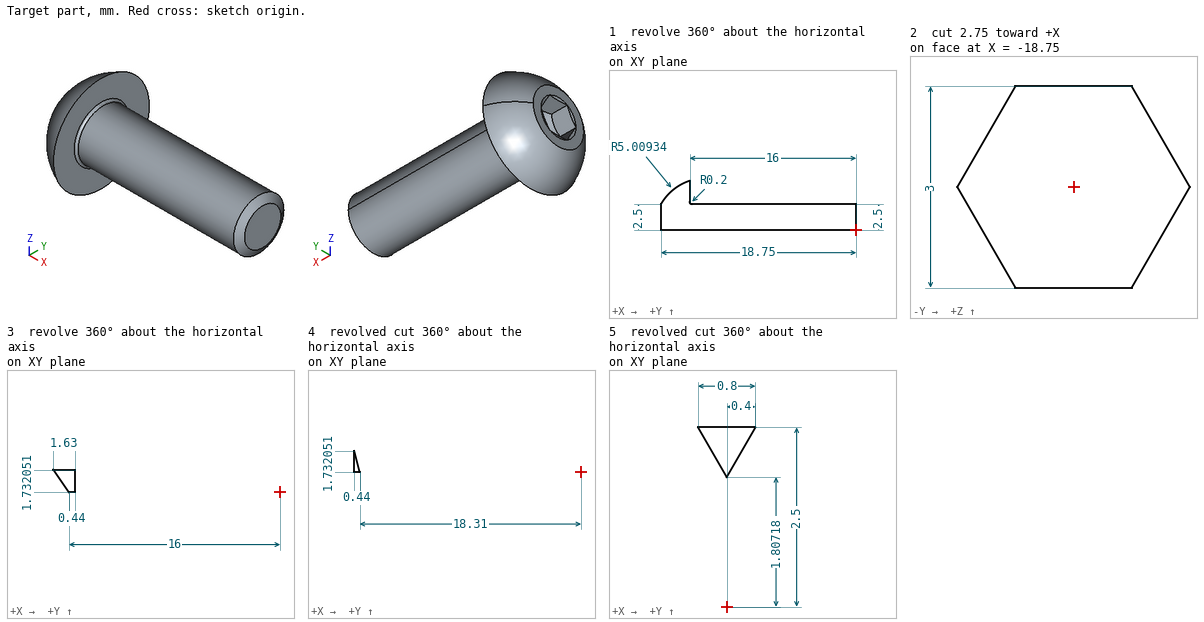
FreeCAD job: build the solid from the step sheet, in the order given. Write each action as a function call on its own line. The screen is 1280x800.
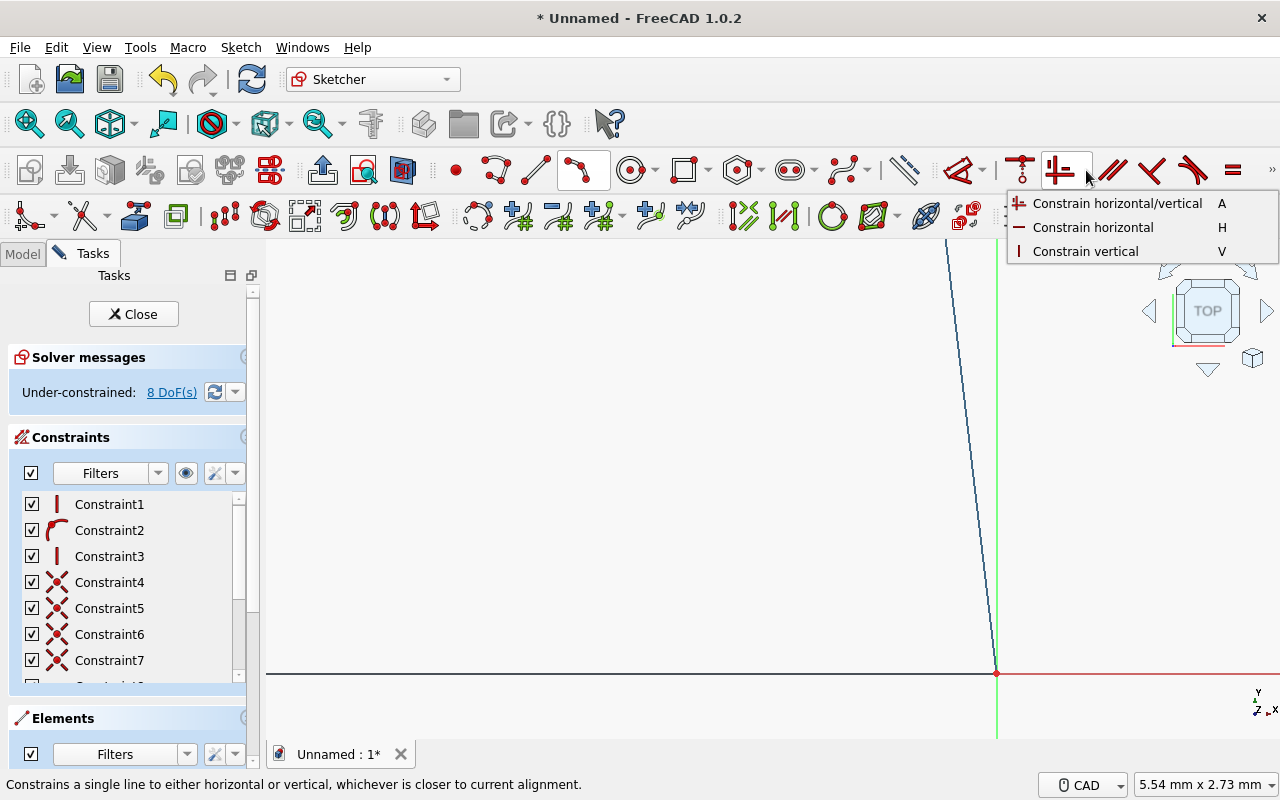
click(1143, 251)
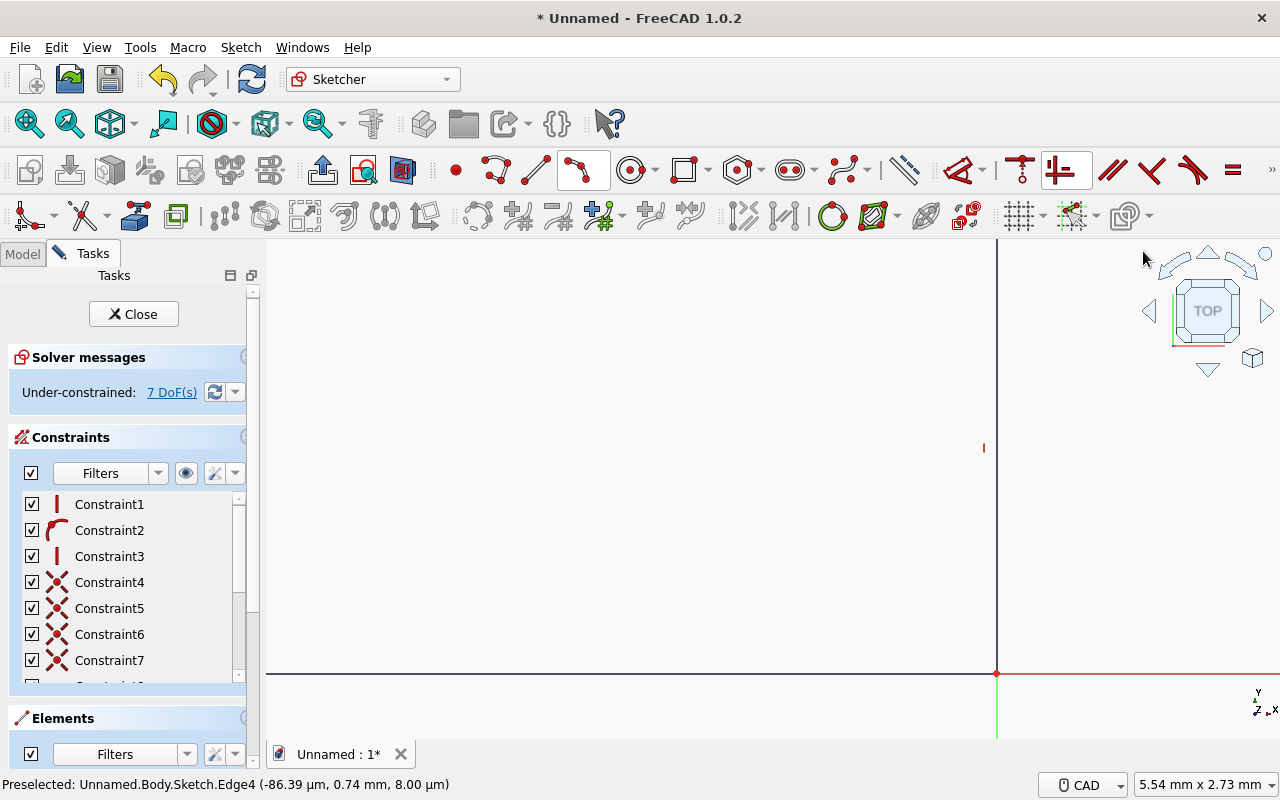
scroll(986, 538, down, 9)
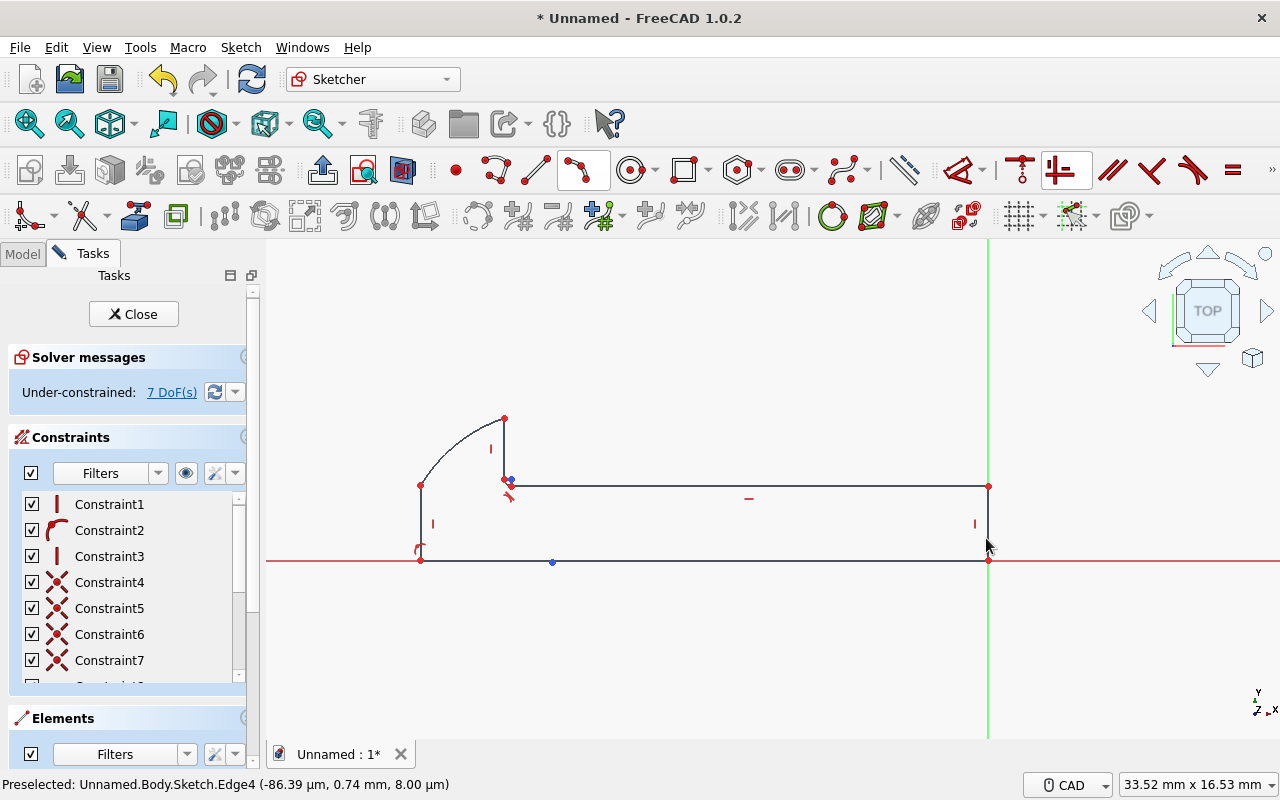
click(552, 563)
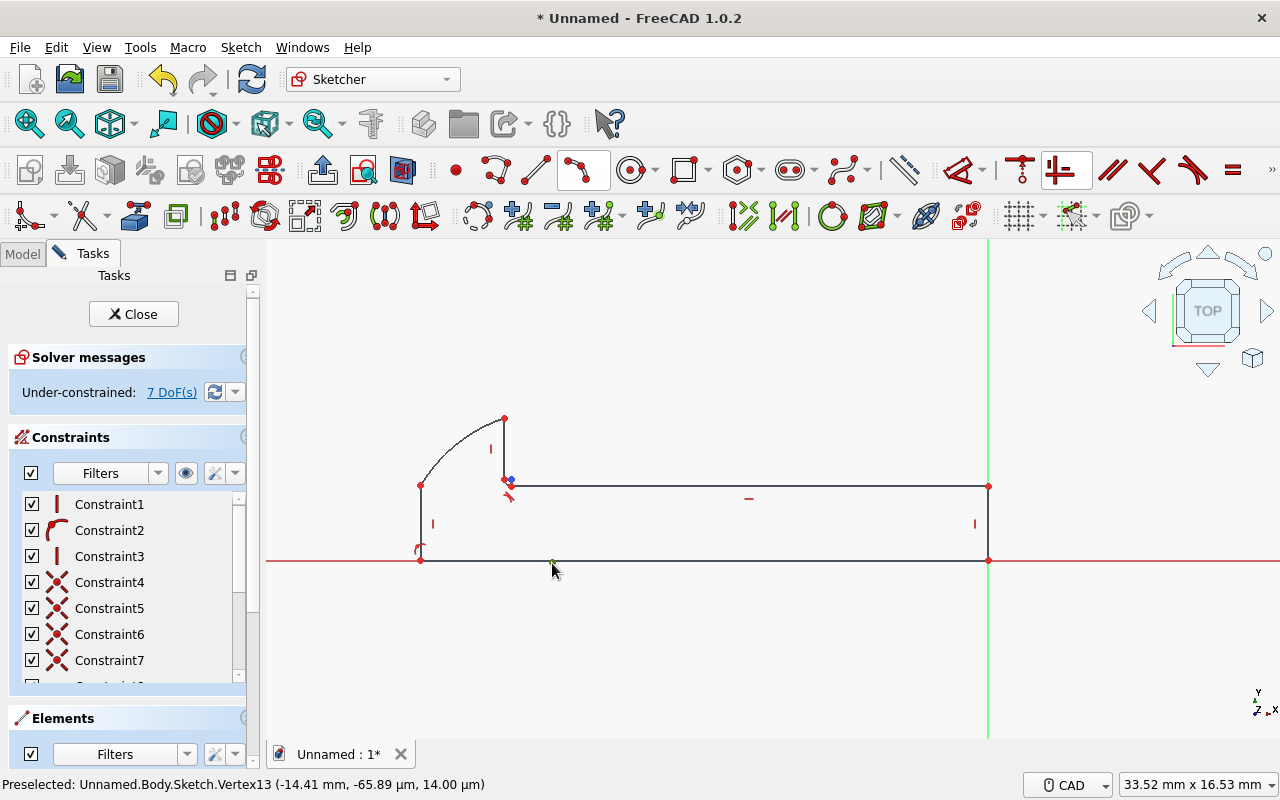
click(353, 561)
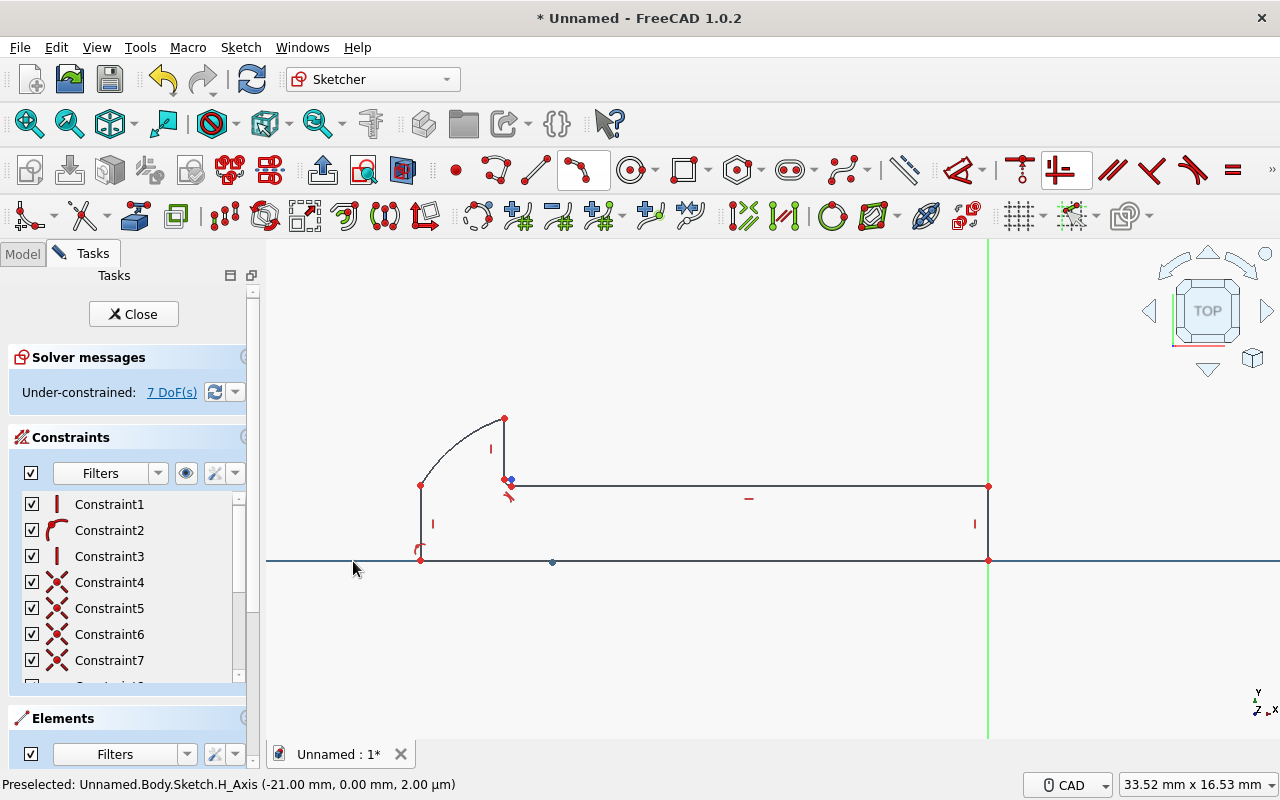
click(1020, 170)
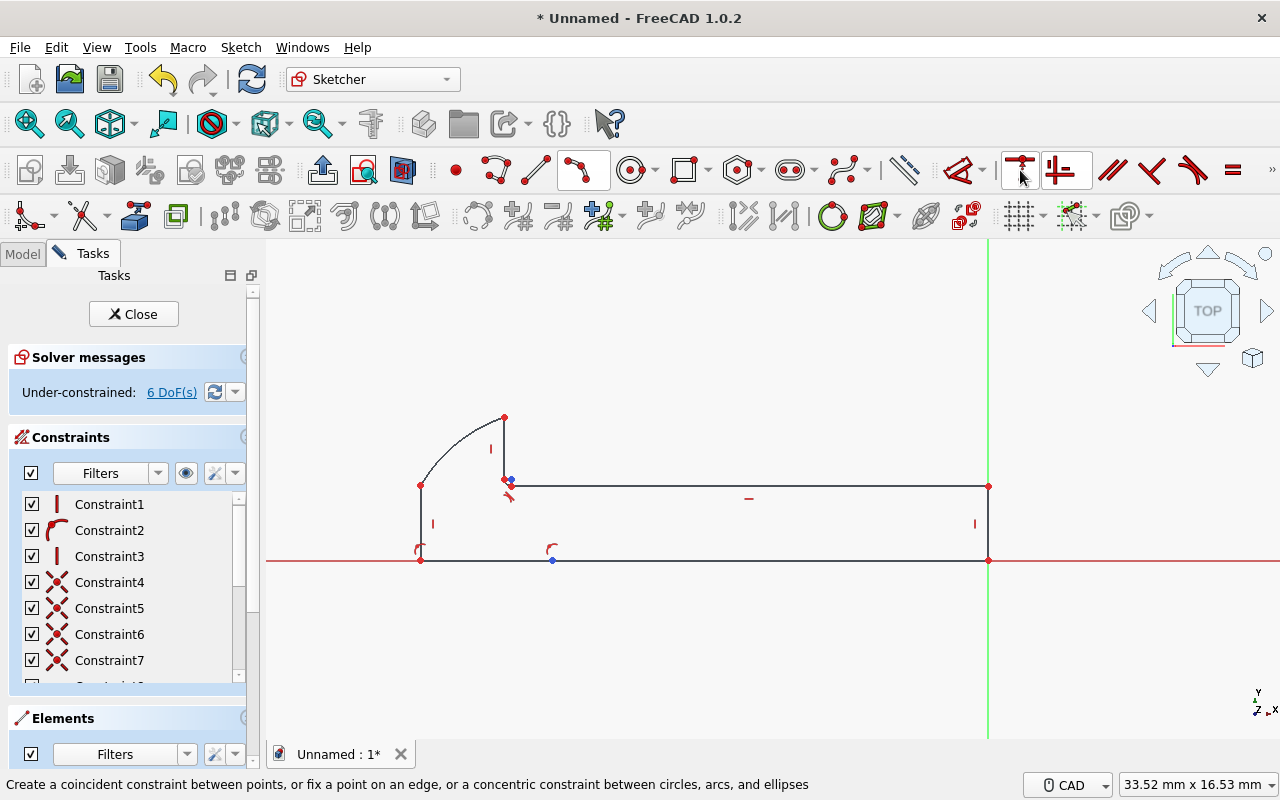
click(474, 431)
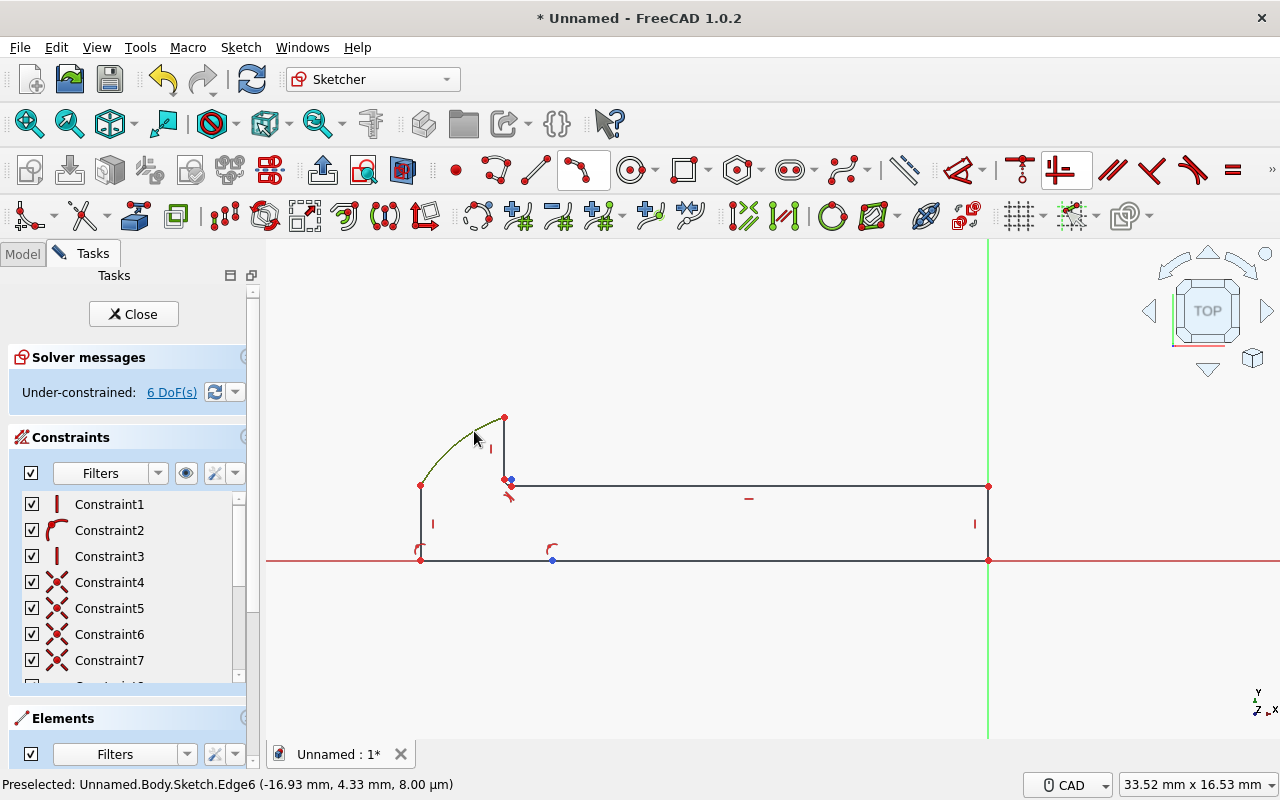
key(k)
key(r)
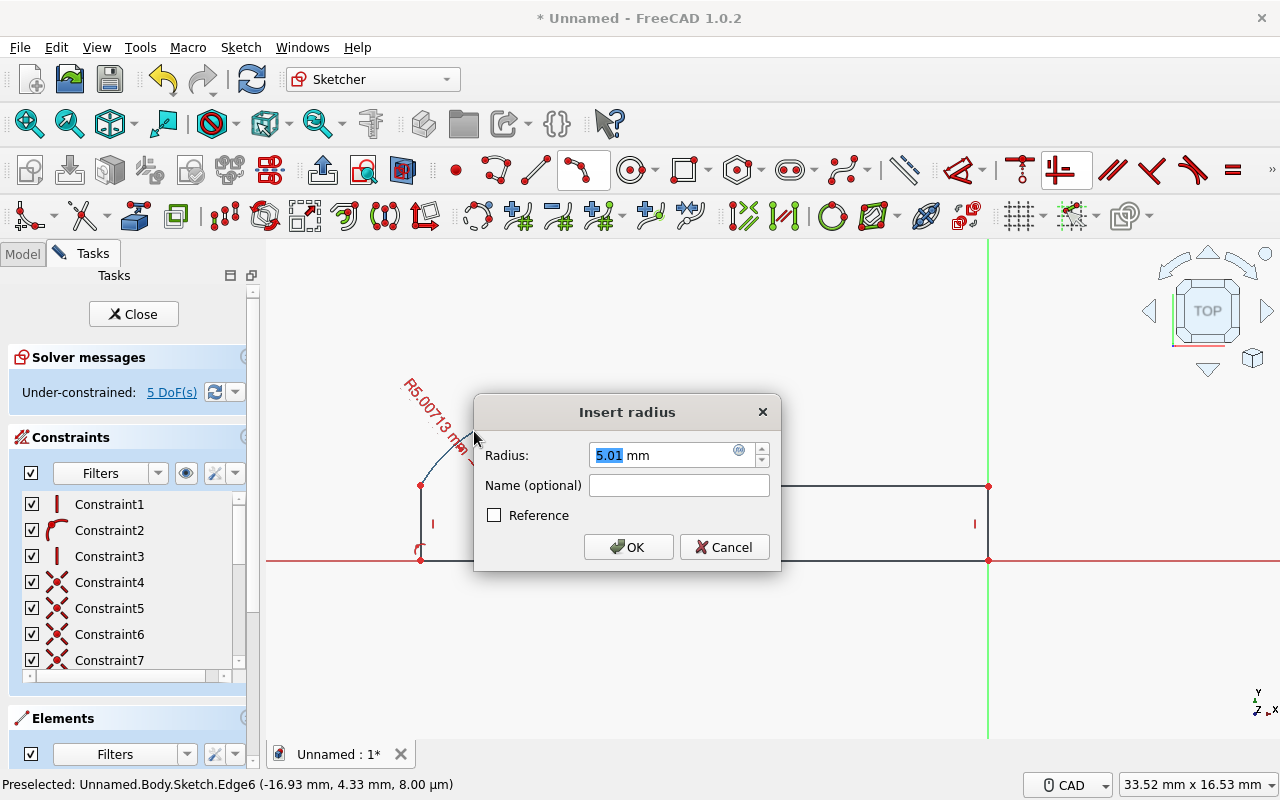
text(5.00934)
key(Return)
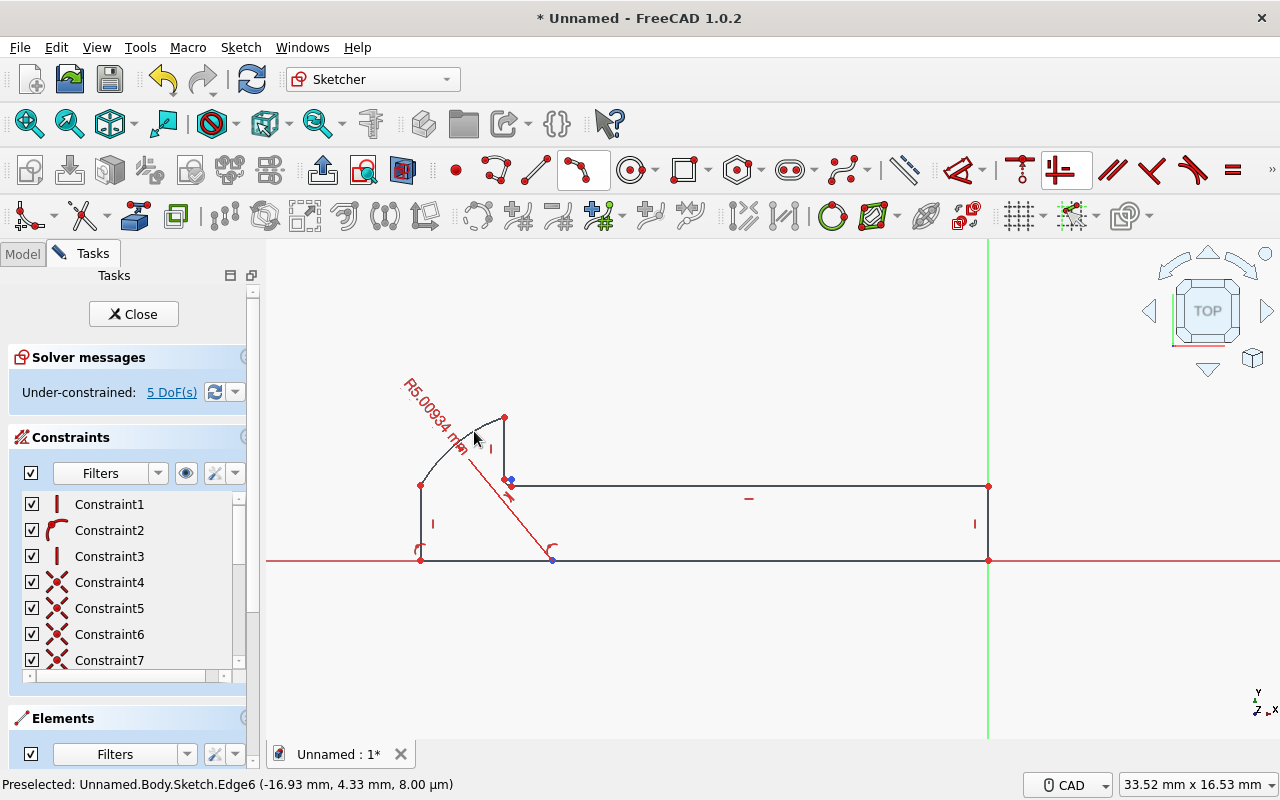
scroll(506, 484, up, 10)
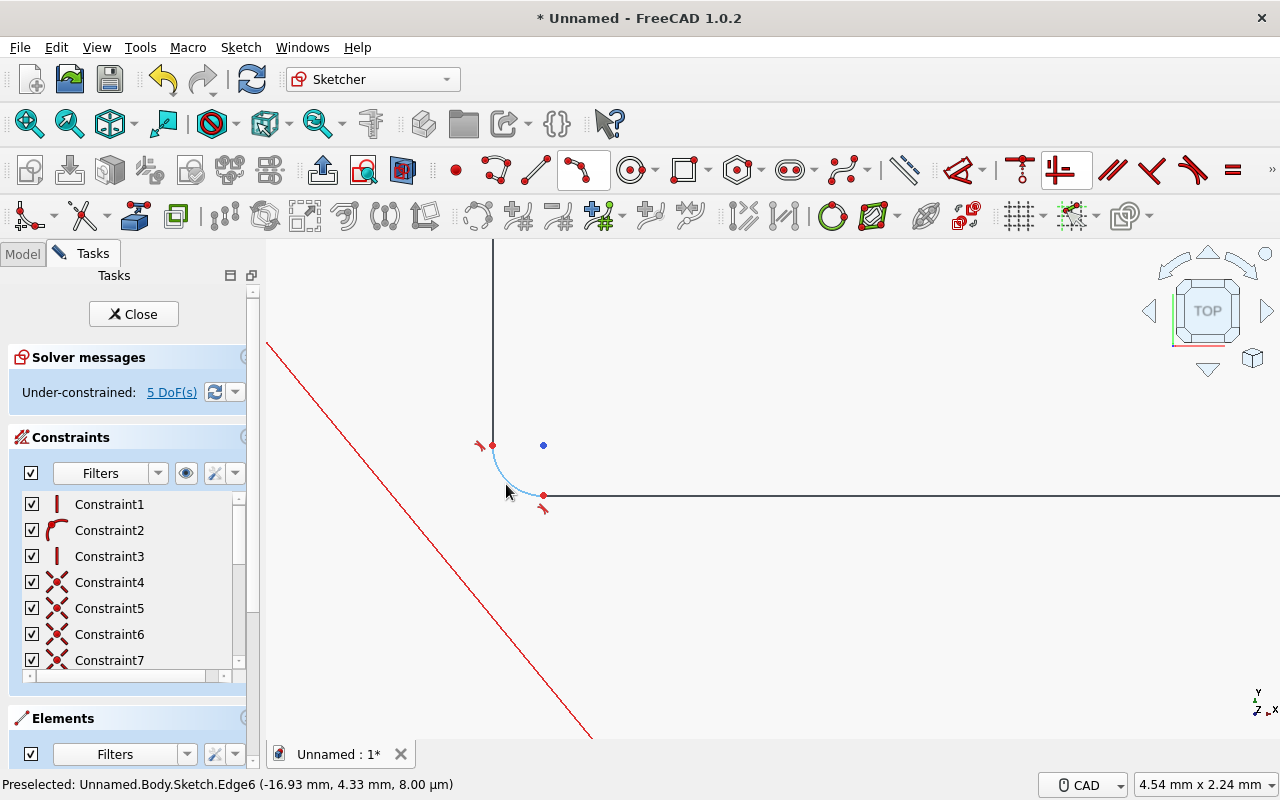
click(508, 481)